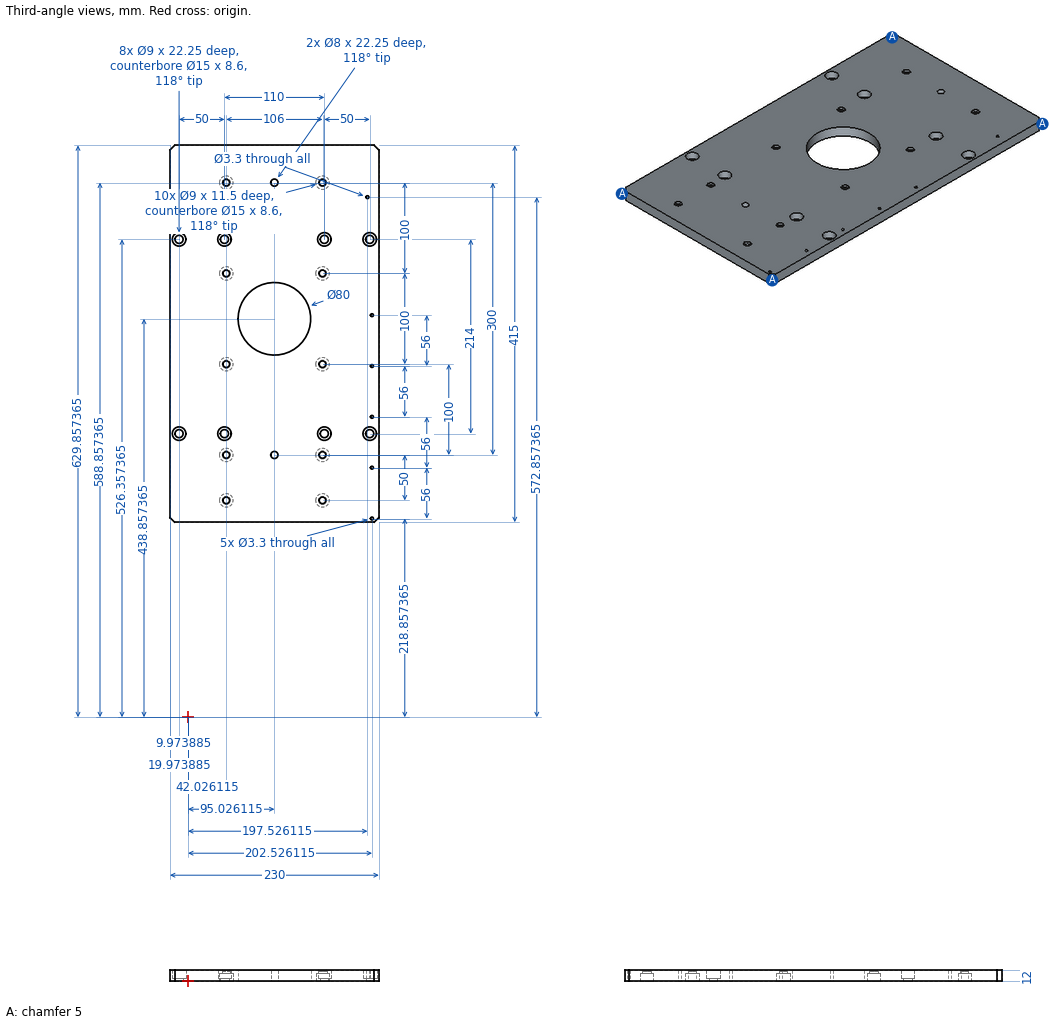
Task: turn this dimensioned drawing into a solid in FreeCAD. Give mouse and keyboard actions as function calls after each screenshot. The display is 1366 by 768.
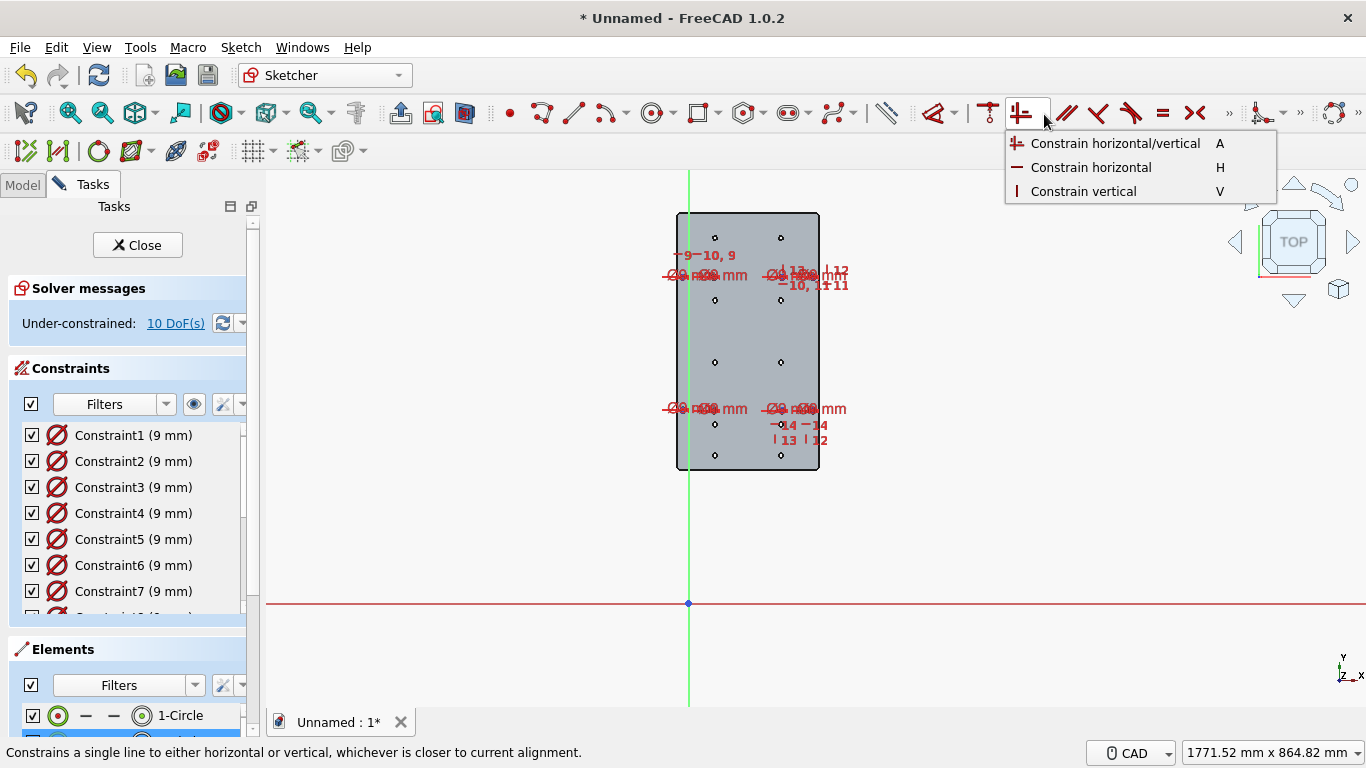
click(1141, 191)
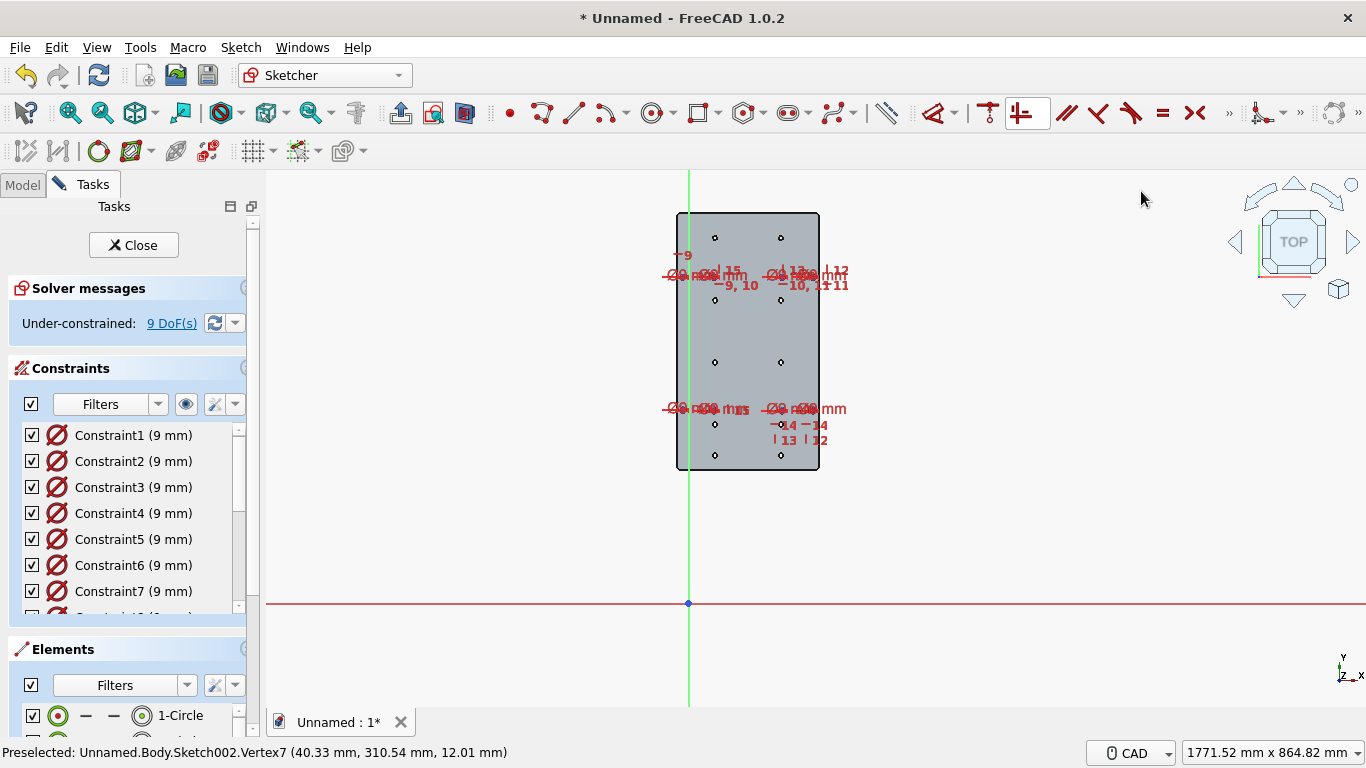
click(782, 411)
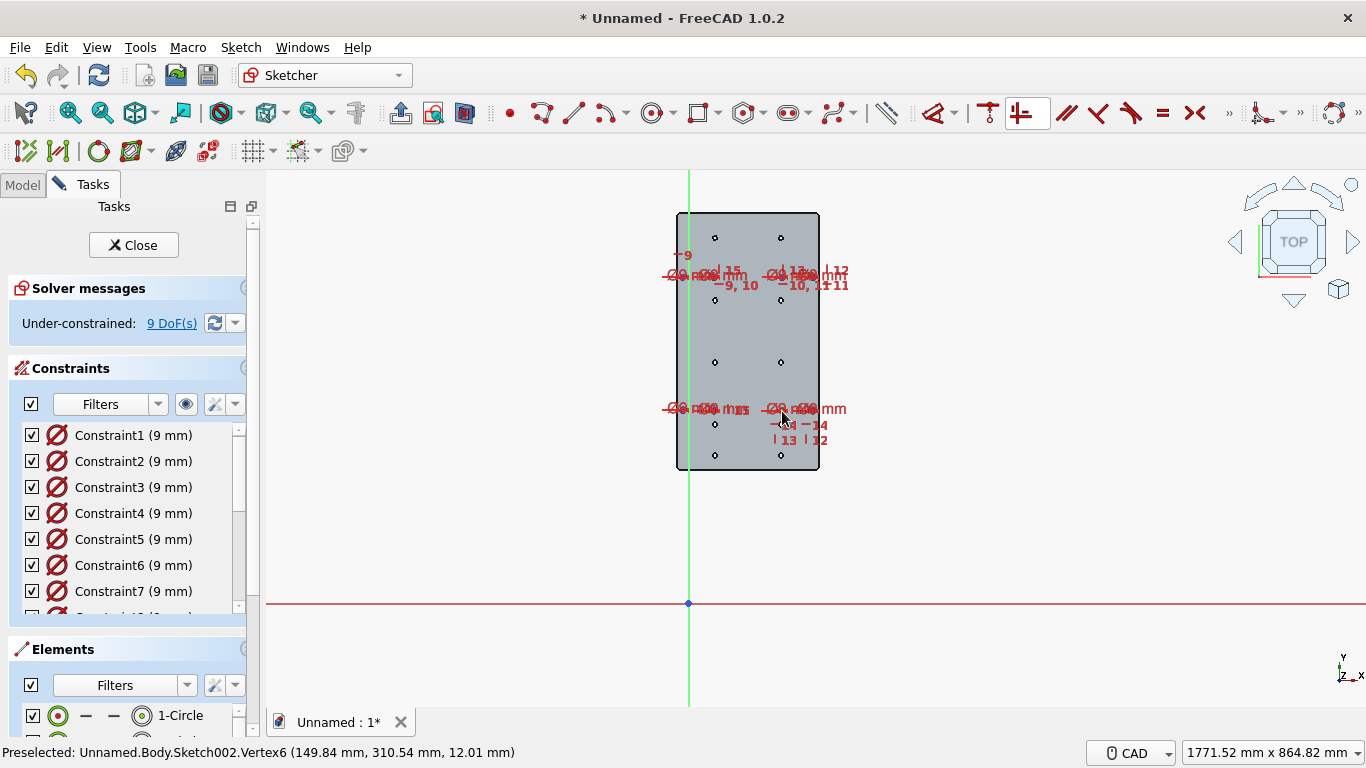
click(714, 411)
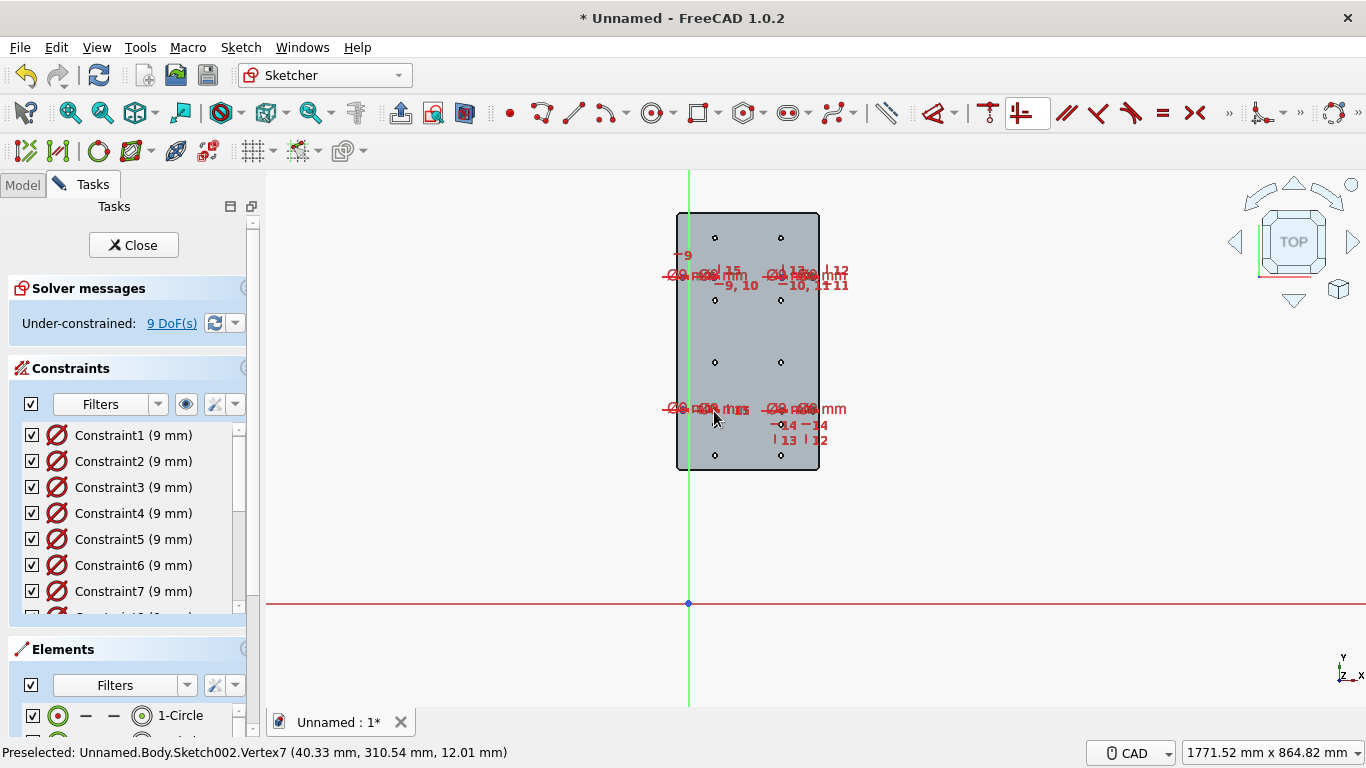
key(h)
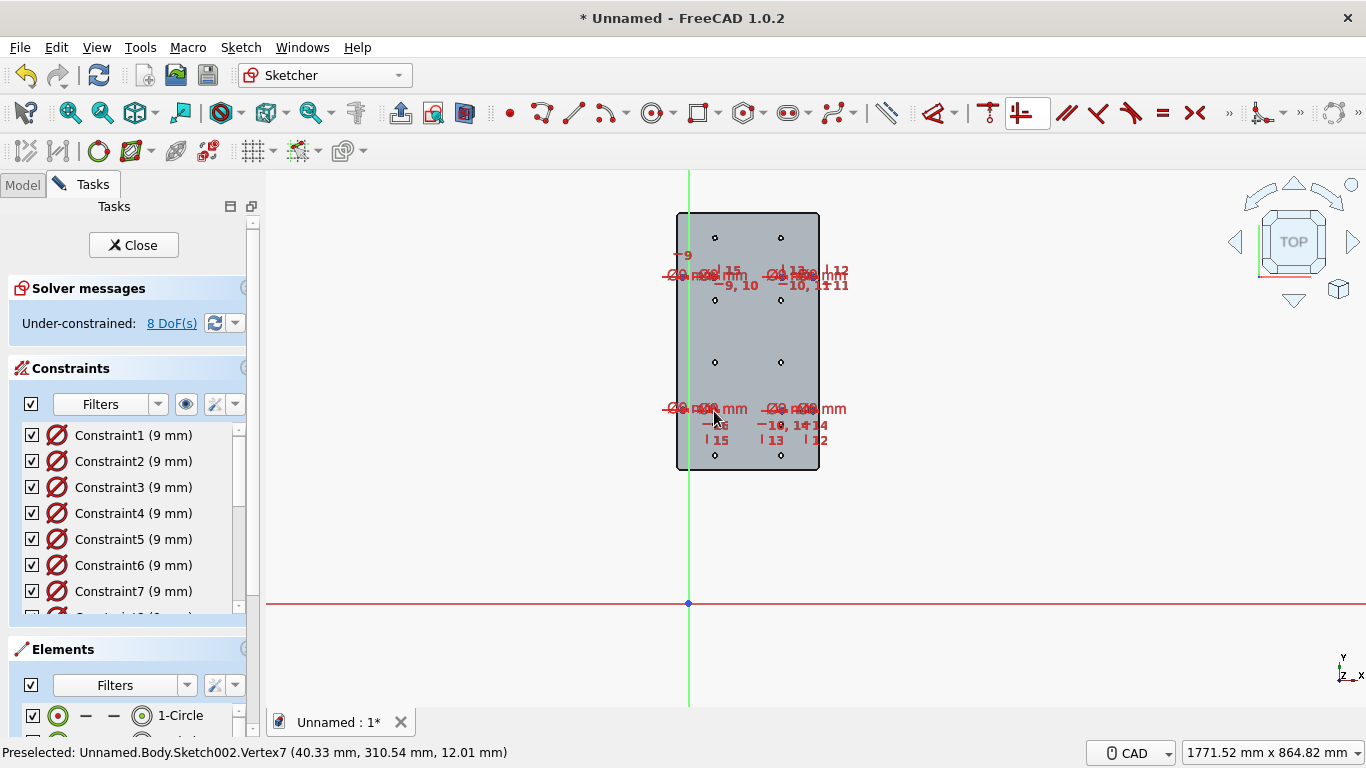
click(683, 277)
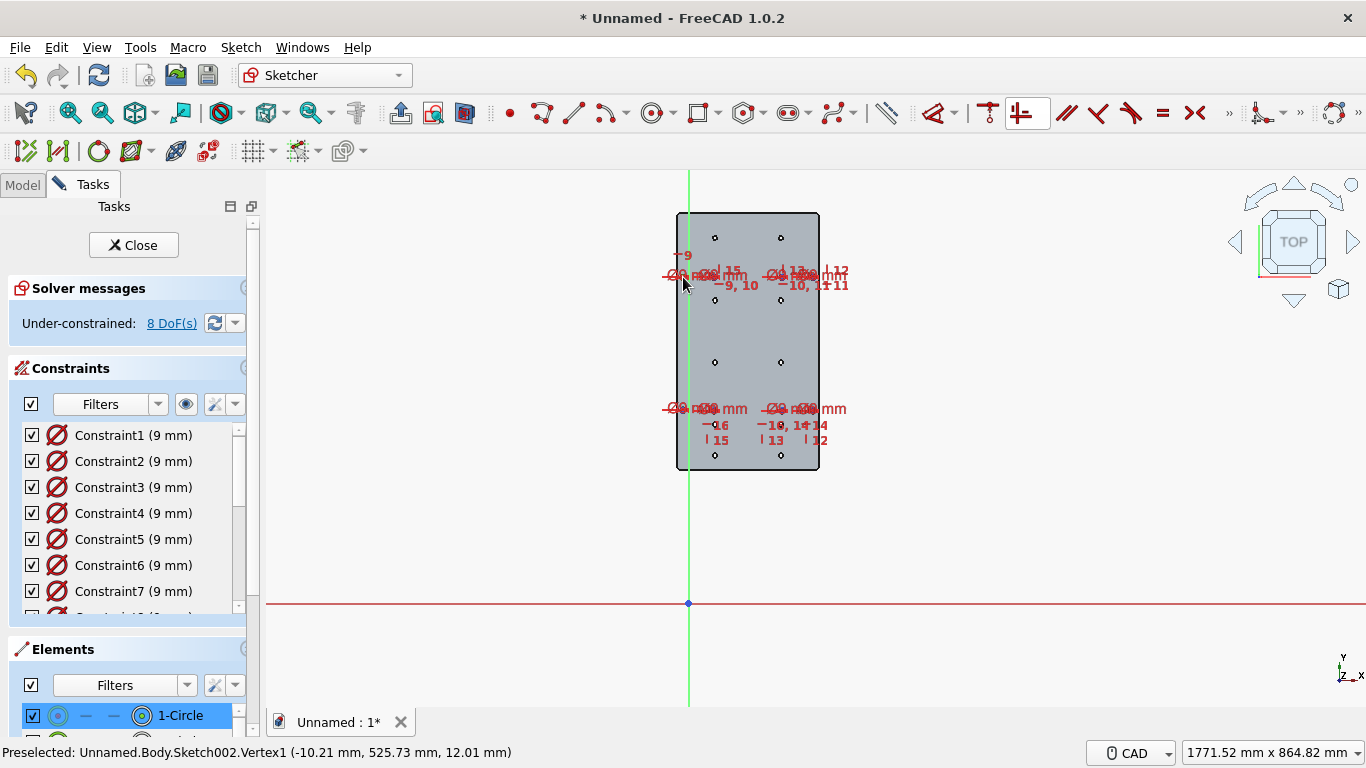
click(683, 410)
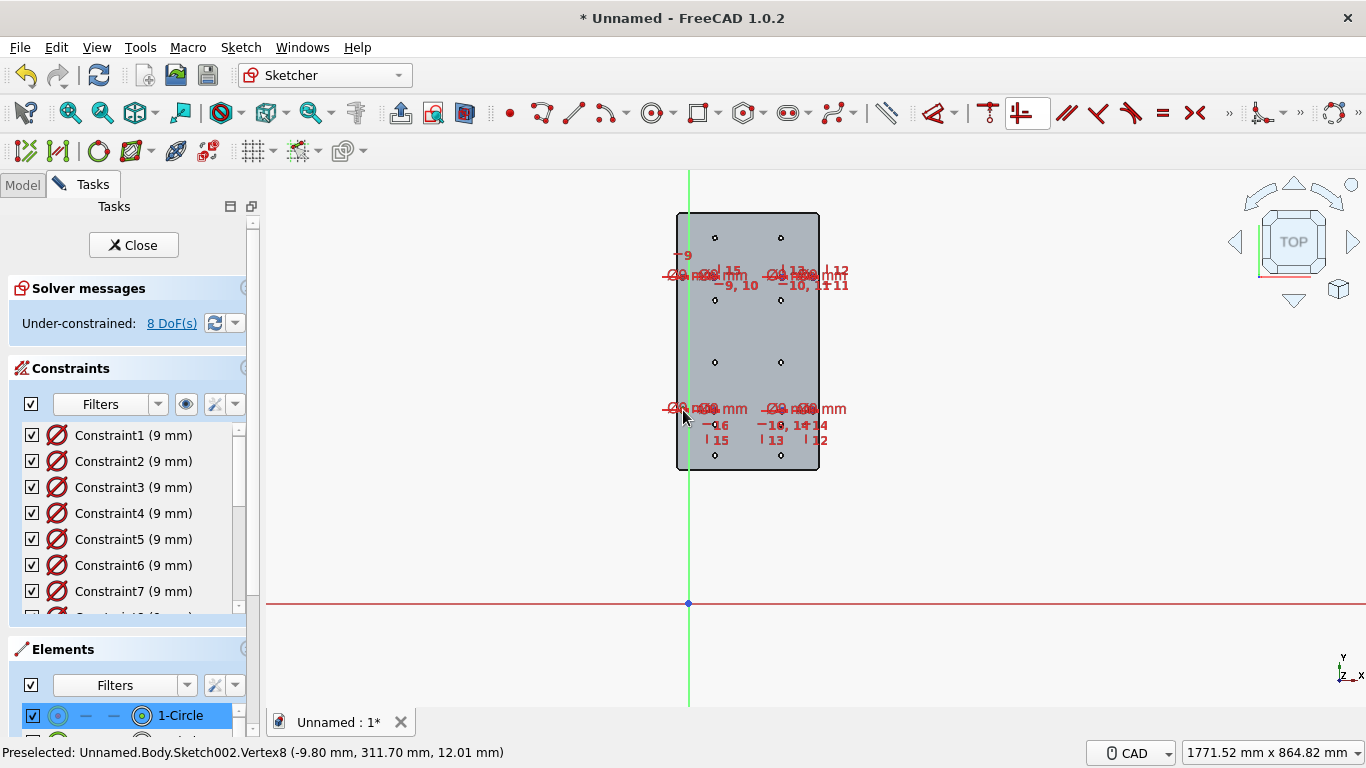
click(1044, 114)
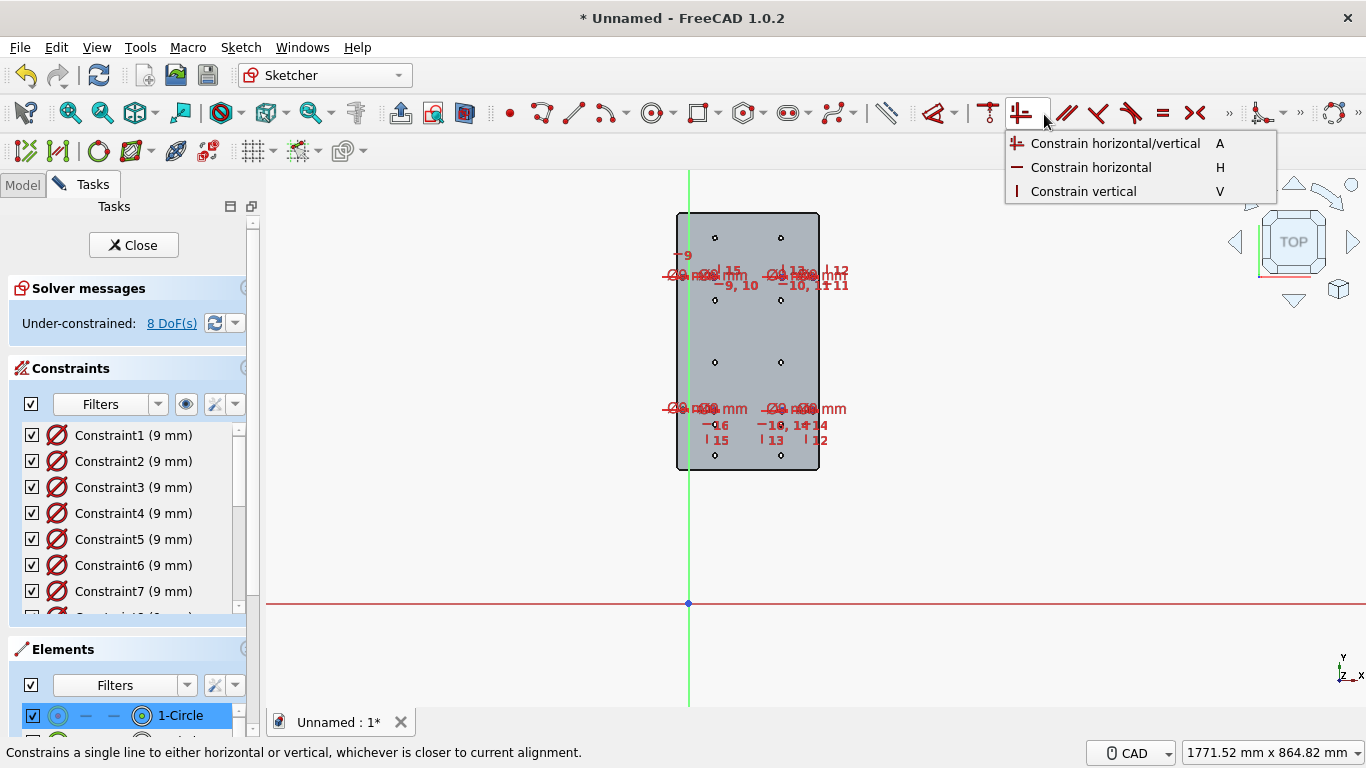
click(1141, 191)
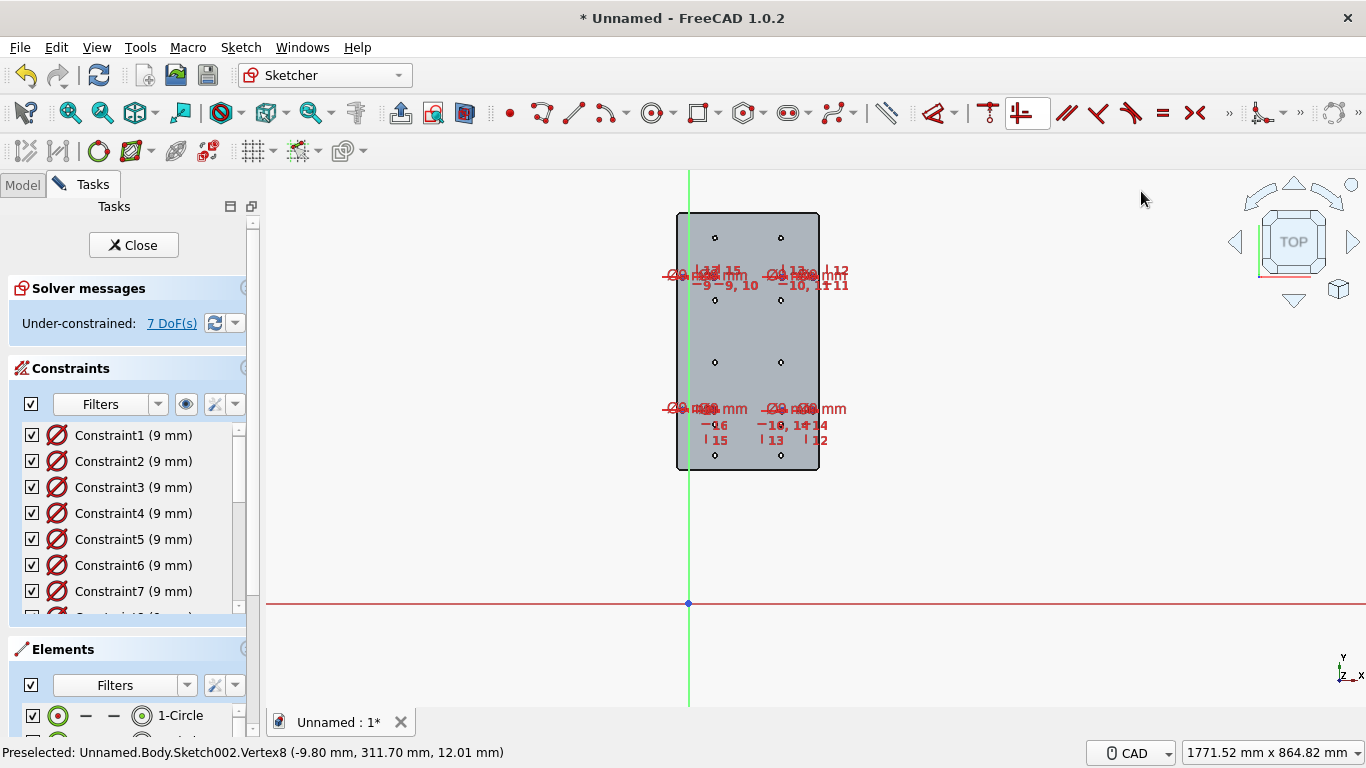
scroll(714, 411, up, 4)